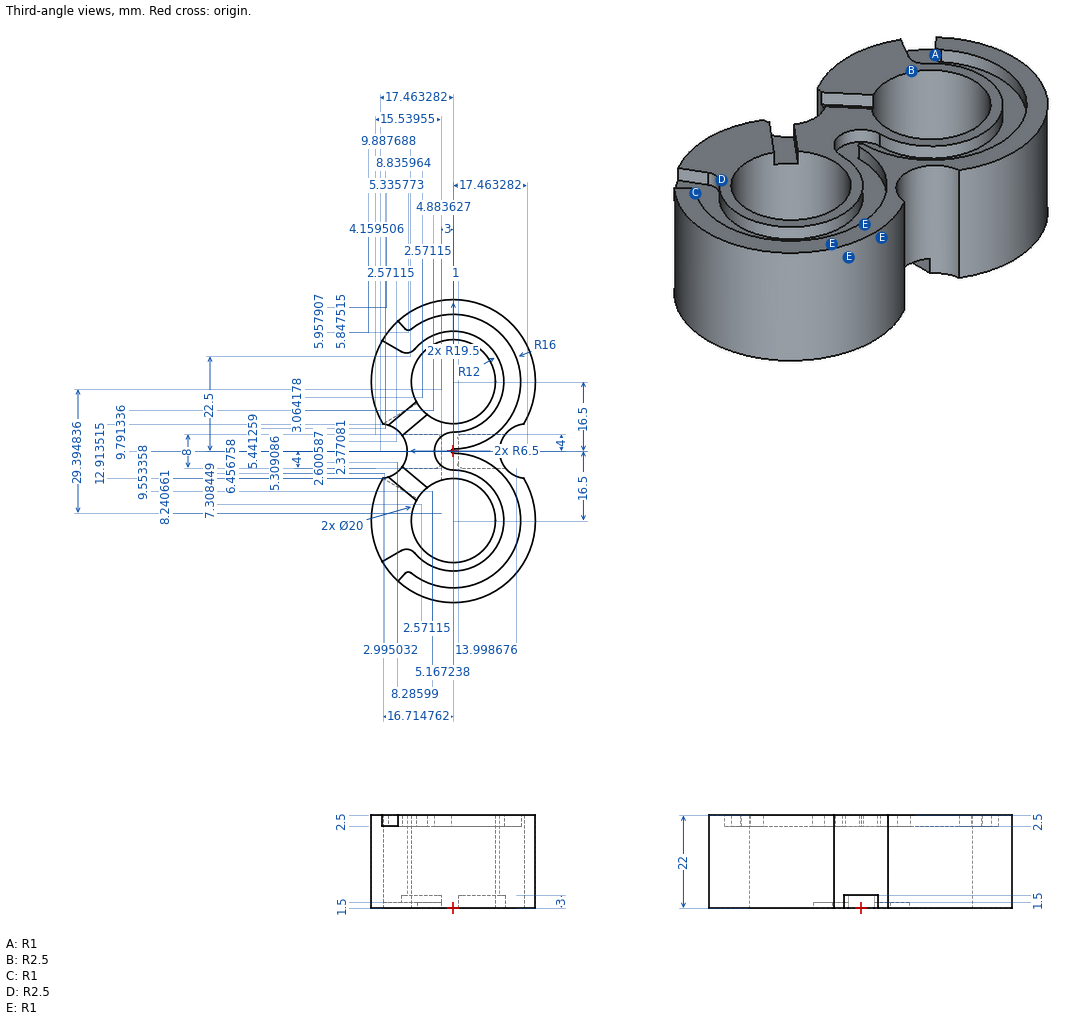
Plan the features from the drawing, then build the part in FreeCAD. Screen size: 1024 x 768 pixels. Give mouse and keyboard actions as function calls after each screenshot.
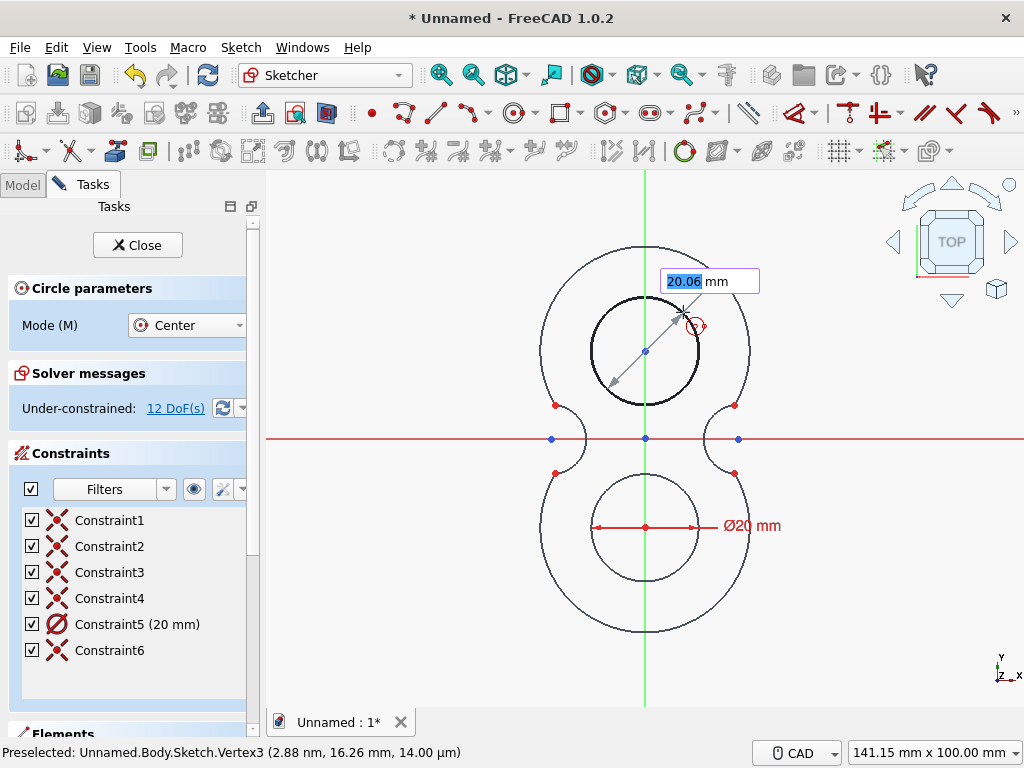
text(20)
key(Return)
key(Escape)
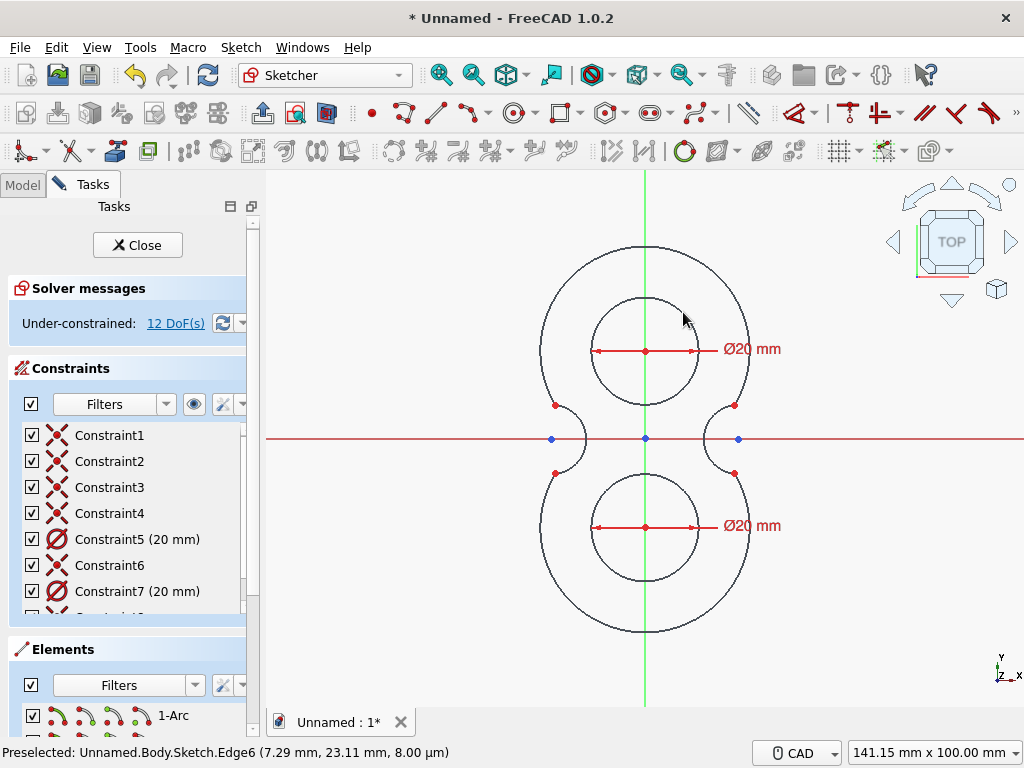
click(723, 282)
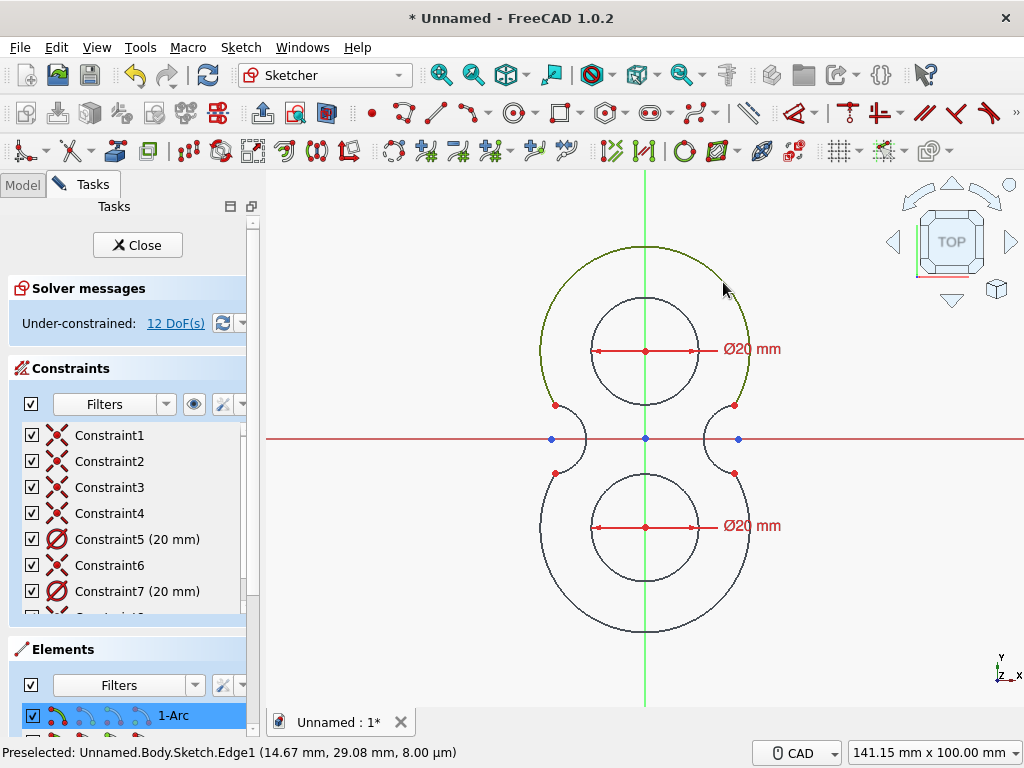
click(567, 597)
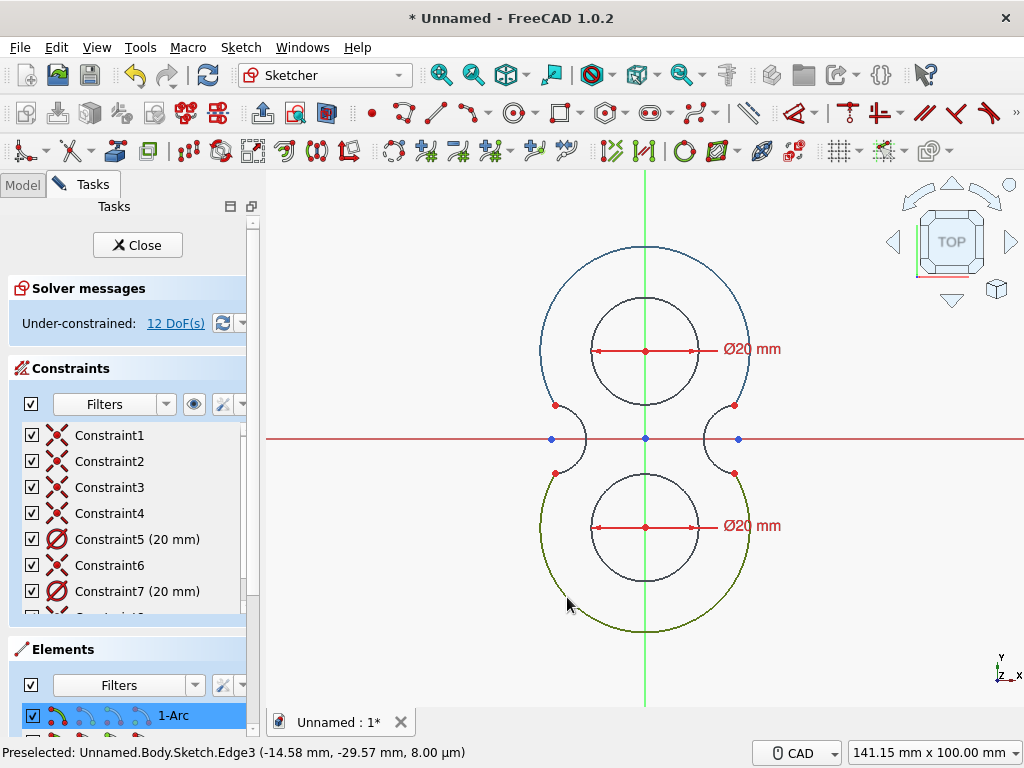
key(e)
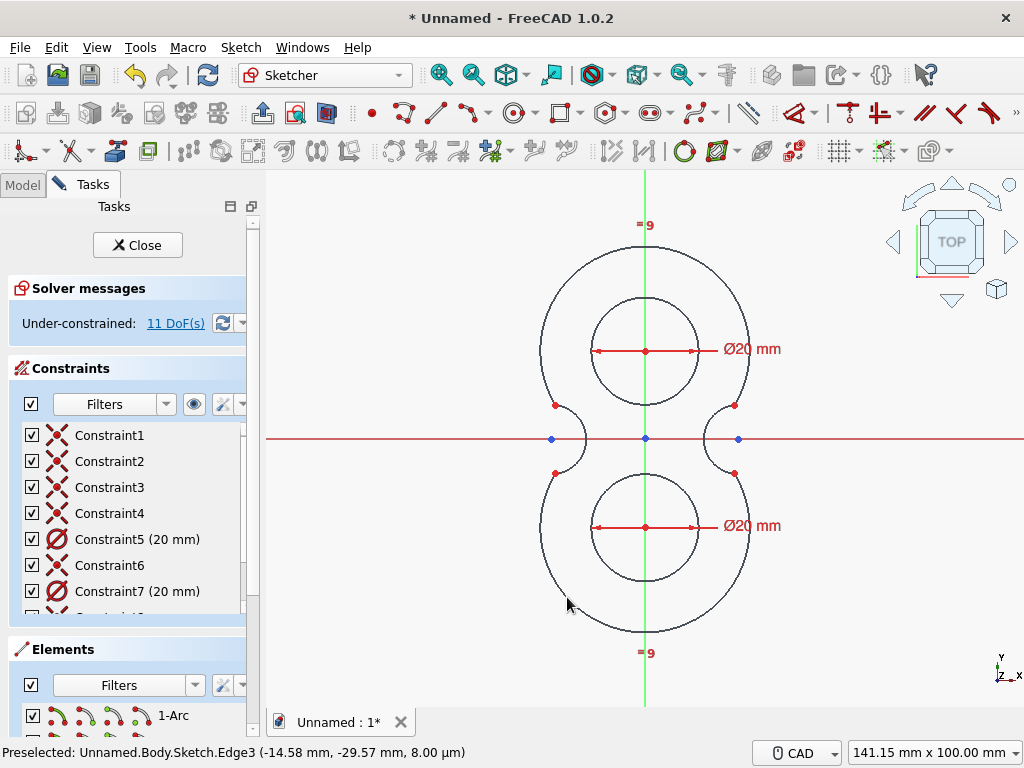
click(580, 459)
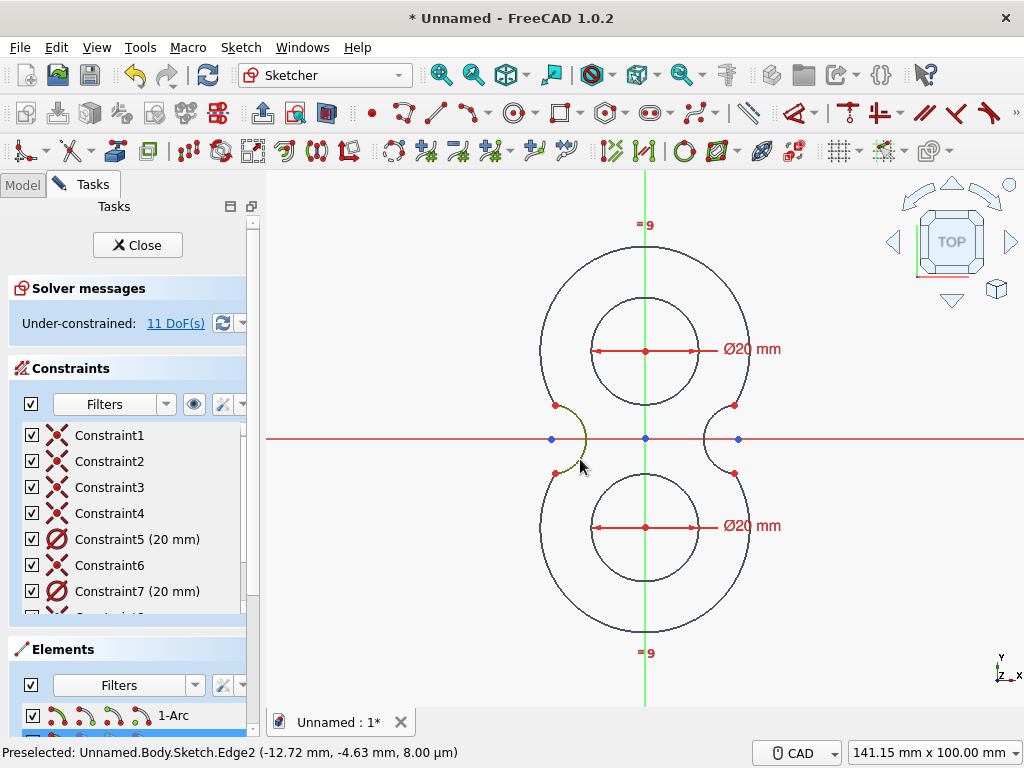
click(710, 420)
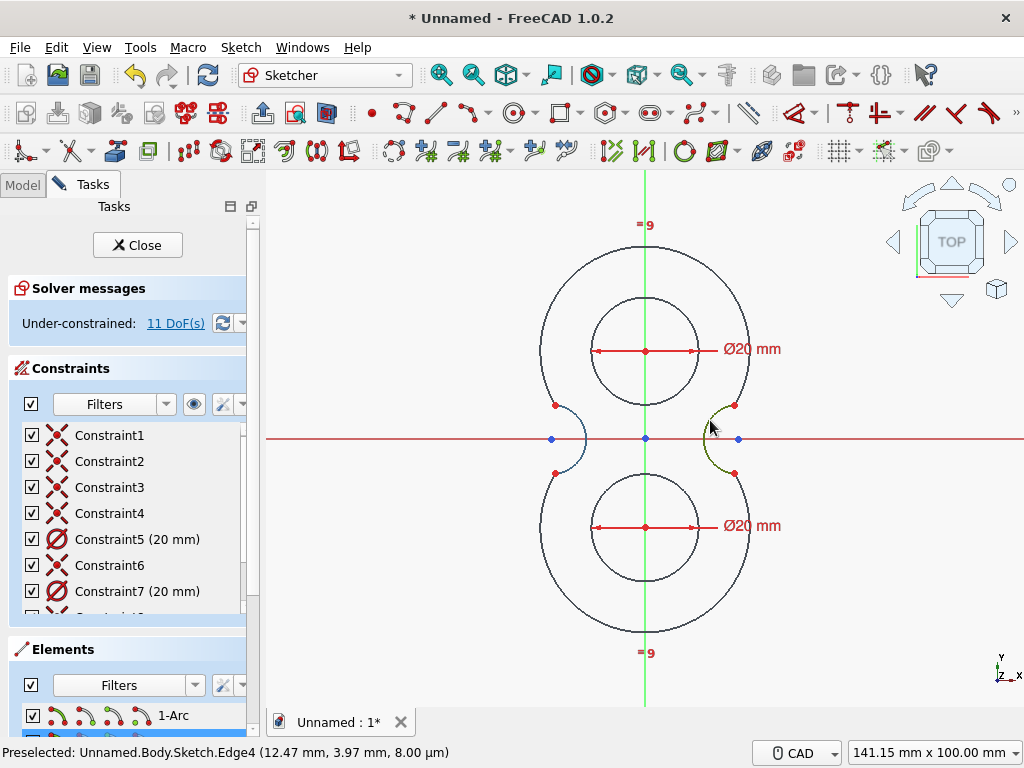
key(e)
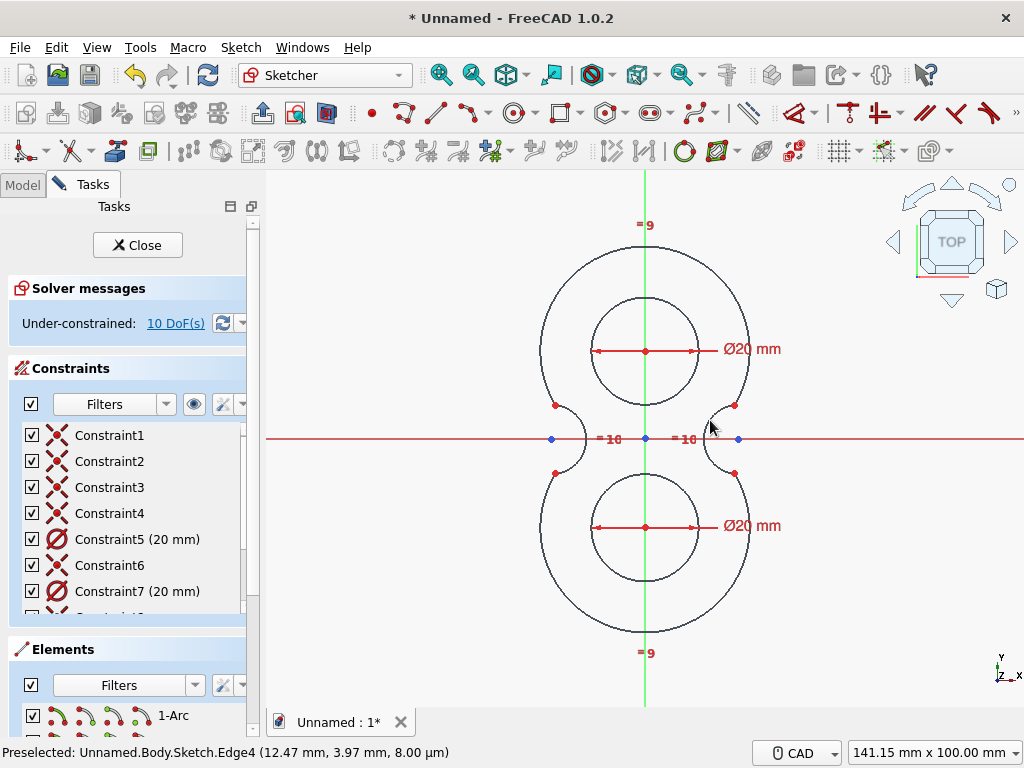
click(645, 351)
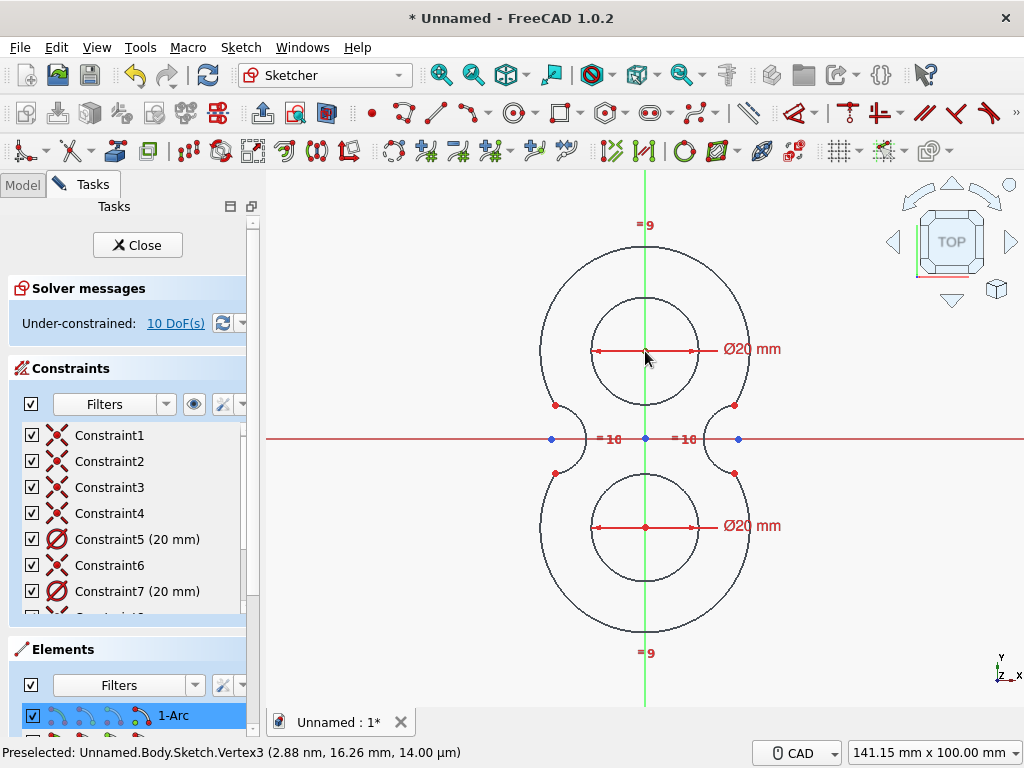
click(645, 542)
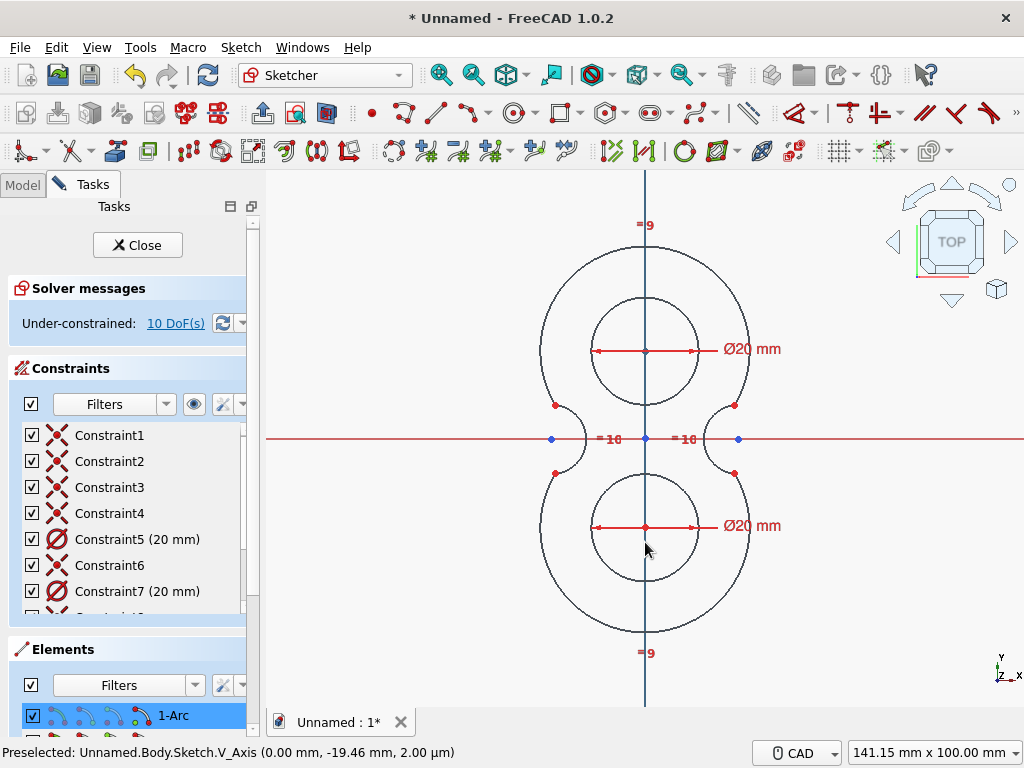
click(848, 114)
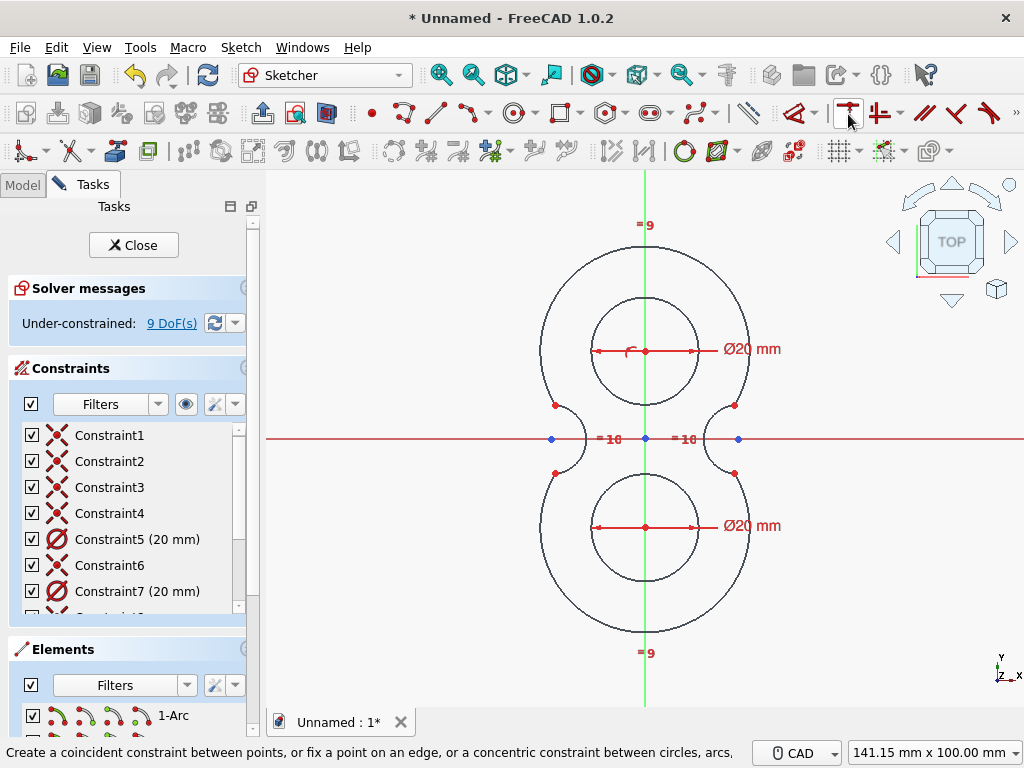
click(552, 439)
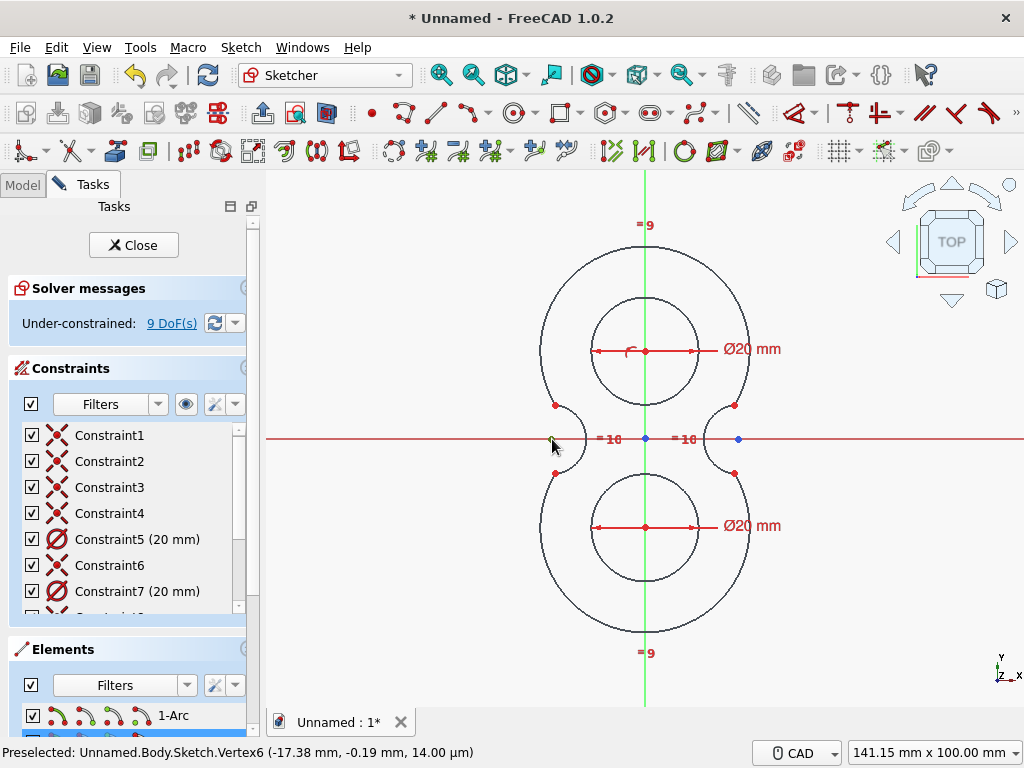
click(334, 438)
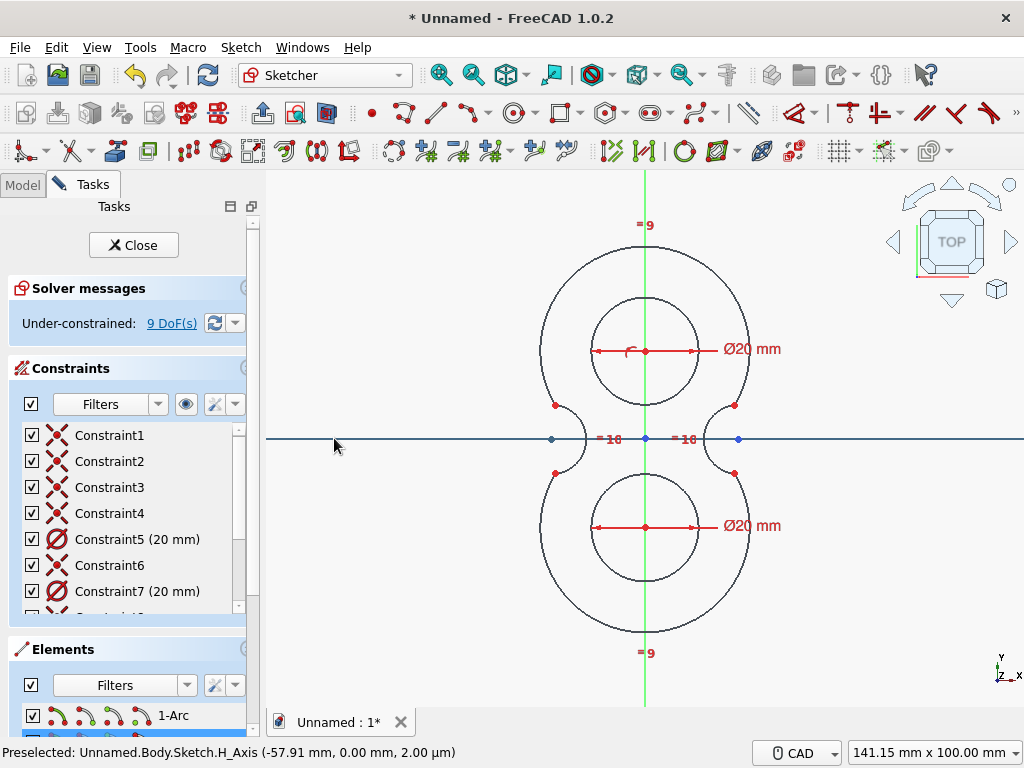
key(c)